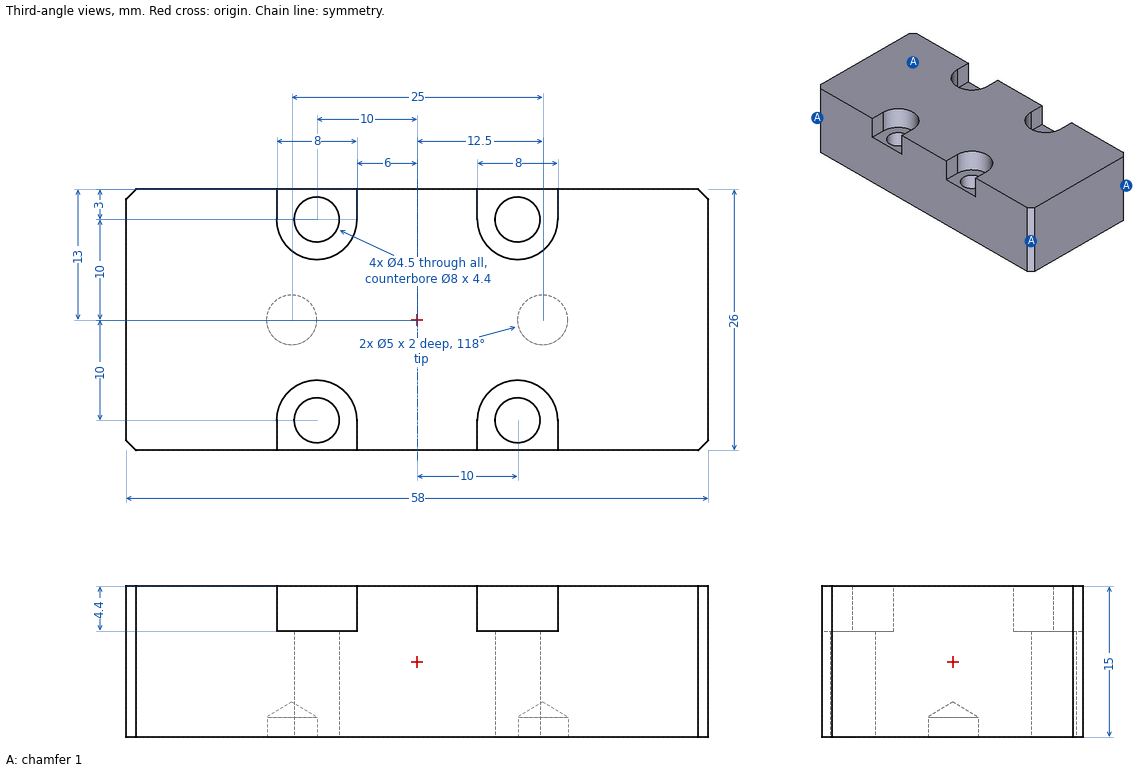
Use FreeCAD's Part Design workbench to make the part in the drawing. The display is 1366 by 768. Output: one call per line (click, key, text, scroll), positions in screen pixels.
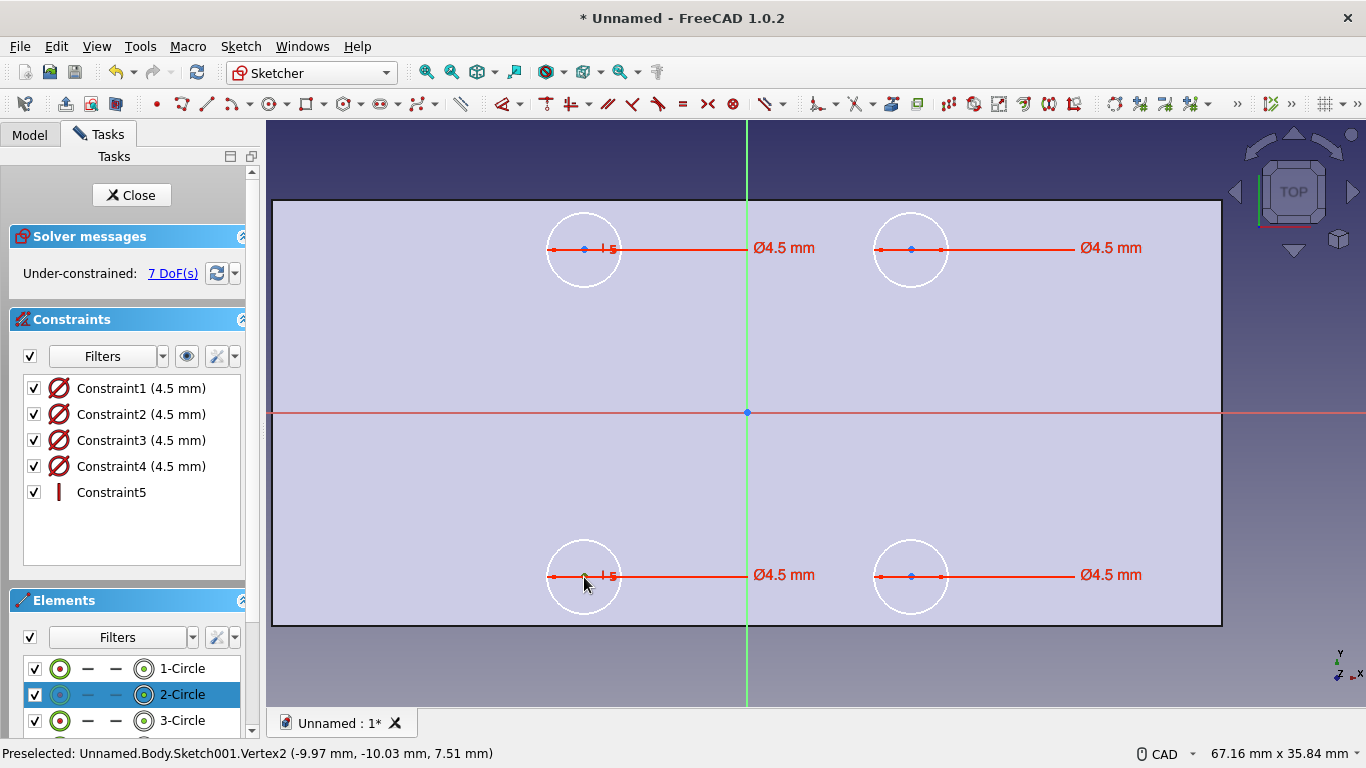
click(911, 577)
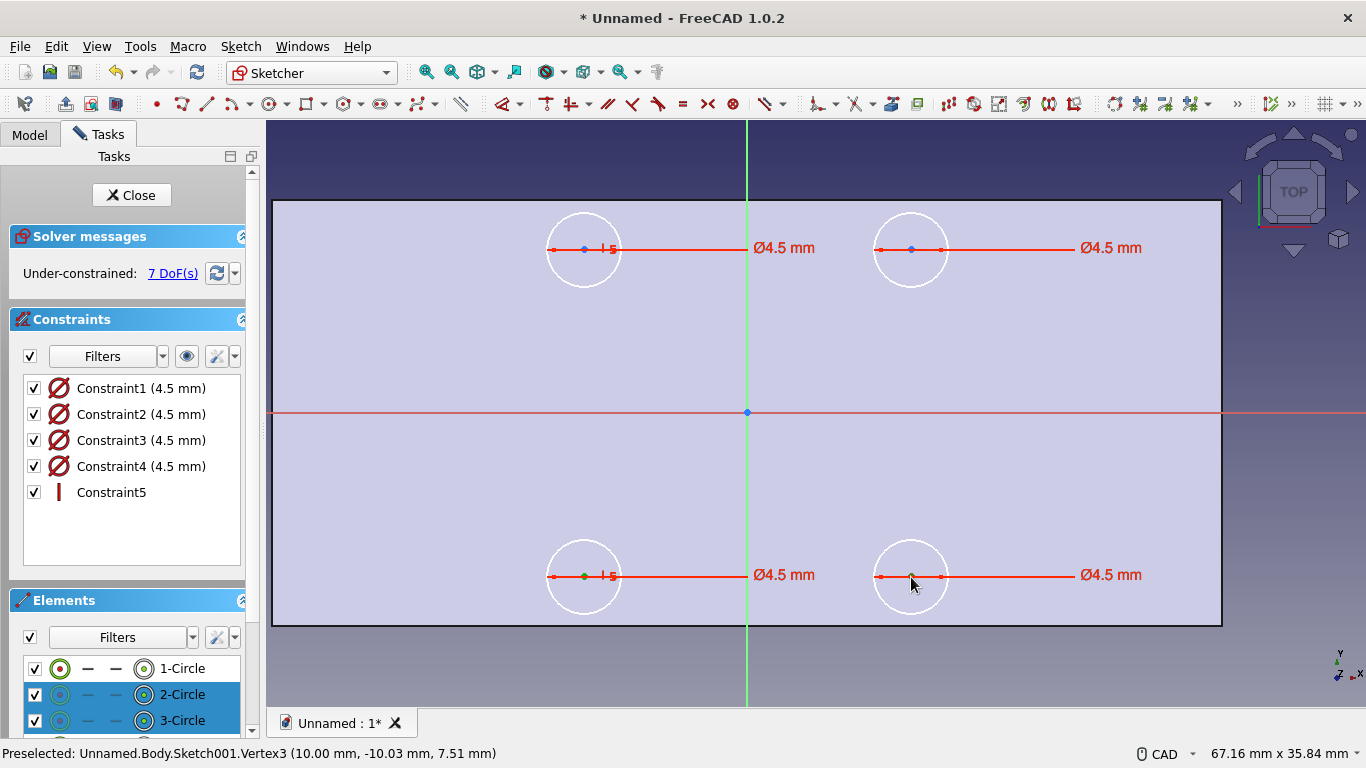
key(h)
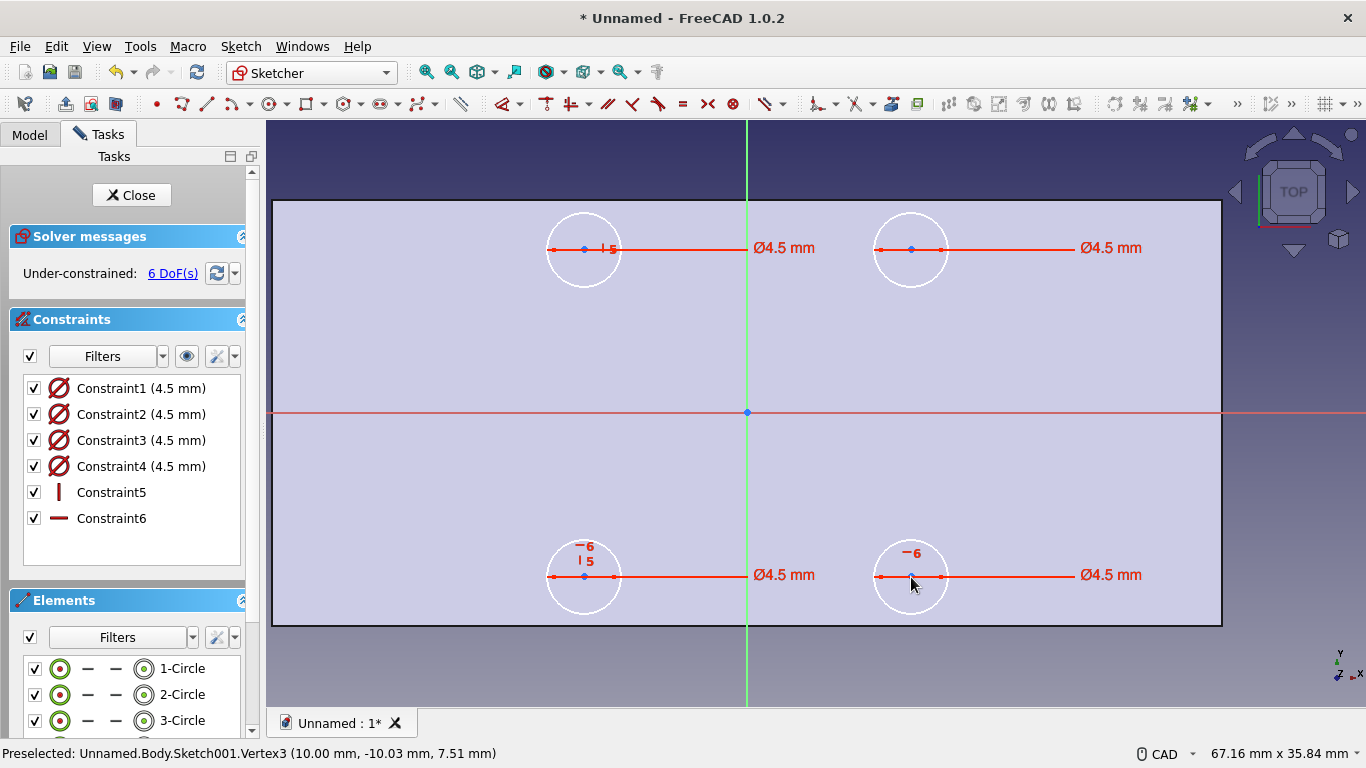
click(911, 577)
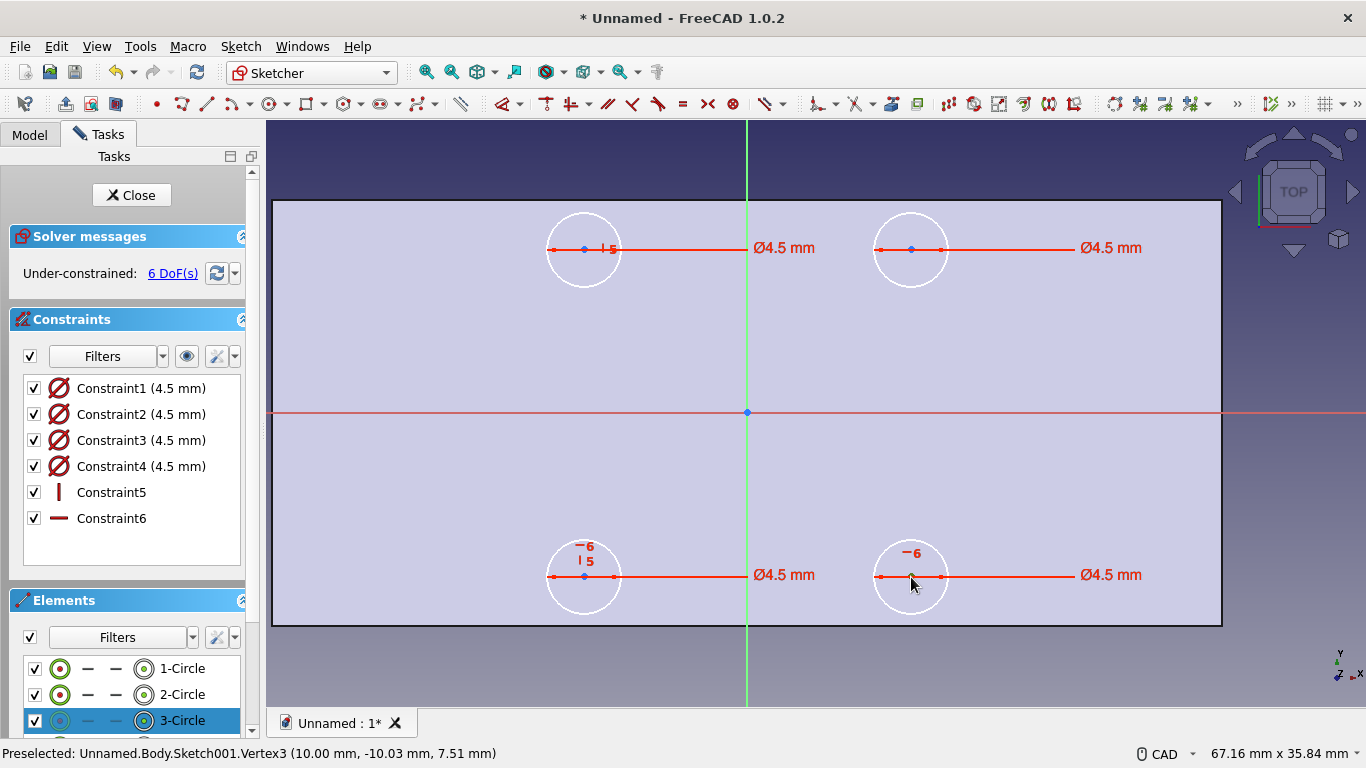
click(911, 250)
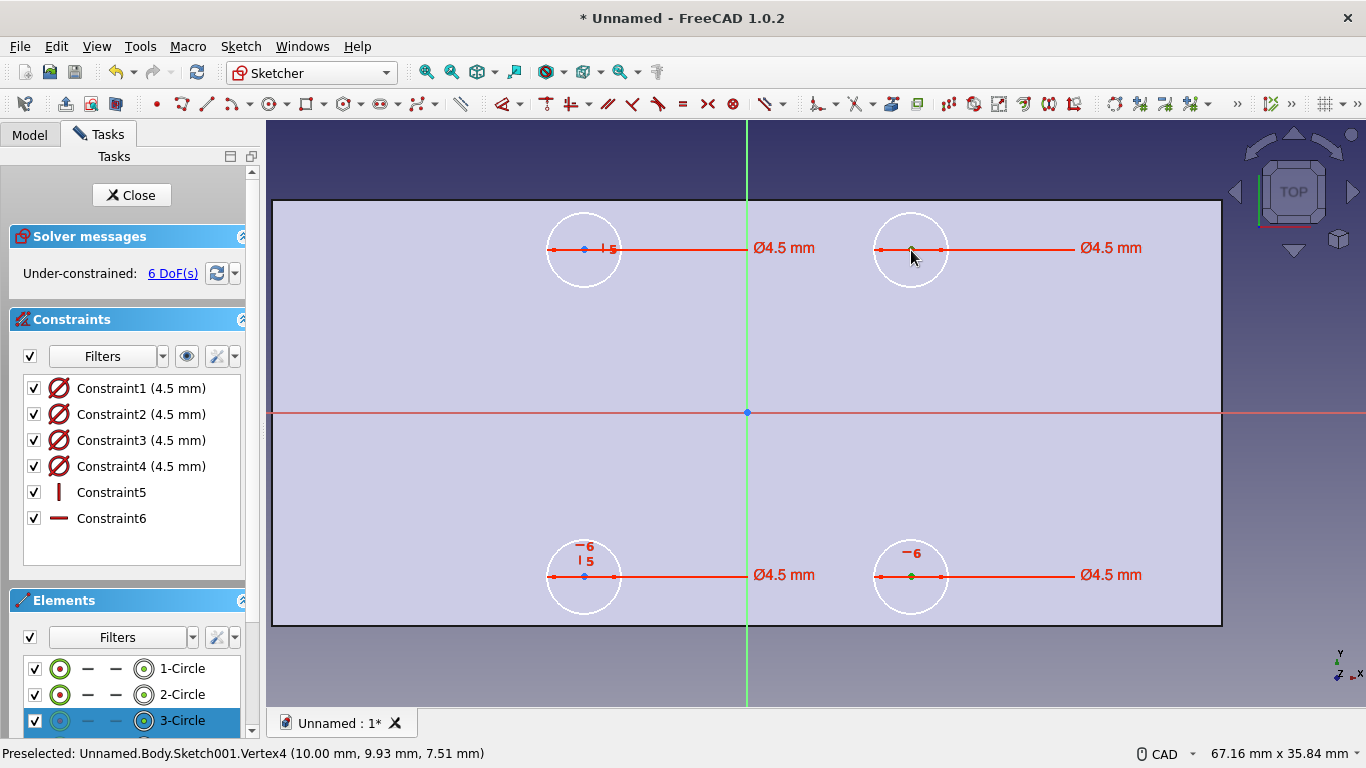
key(v)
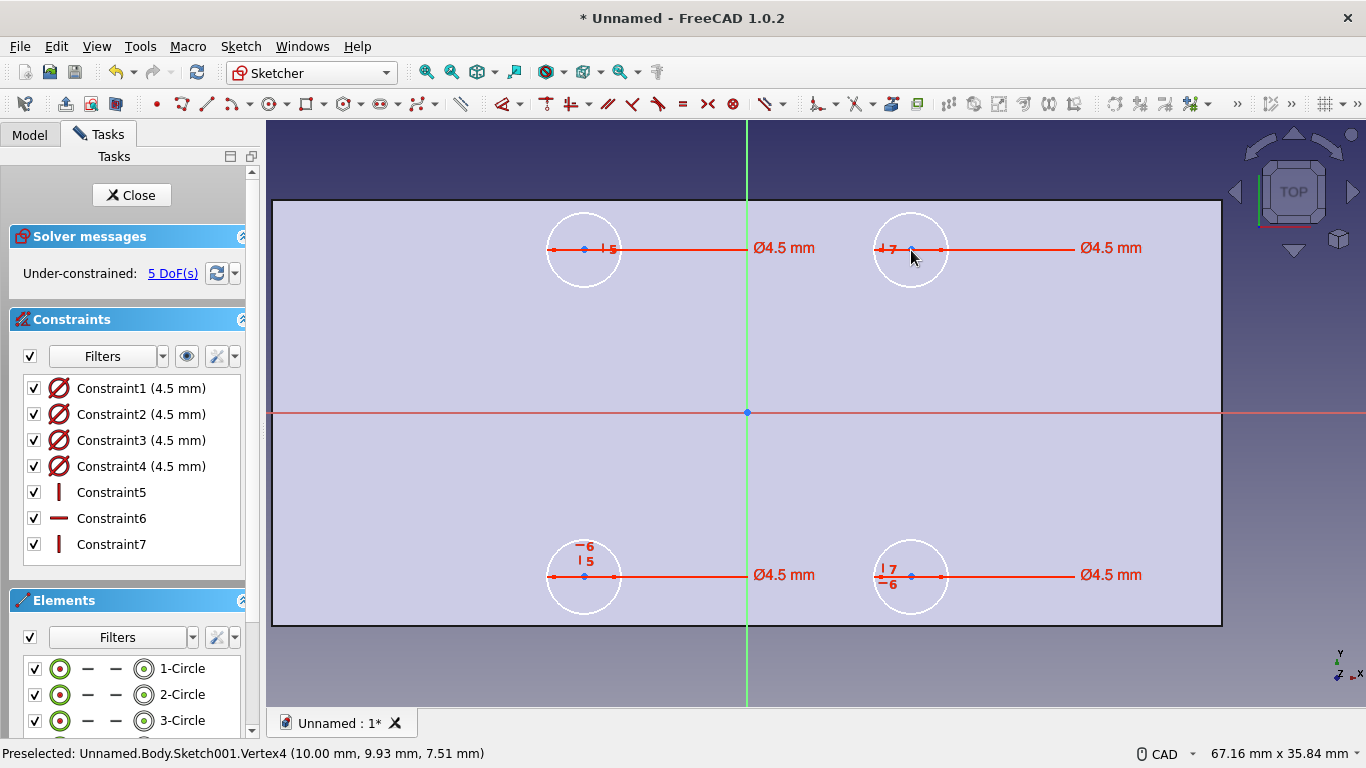
click(584, 250)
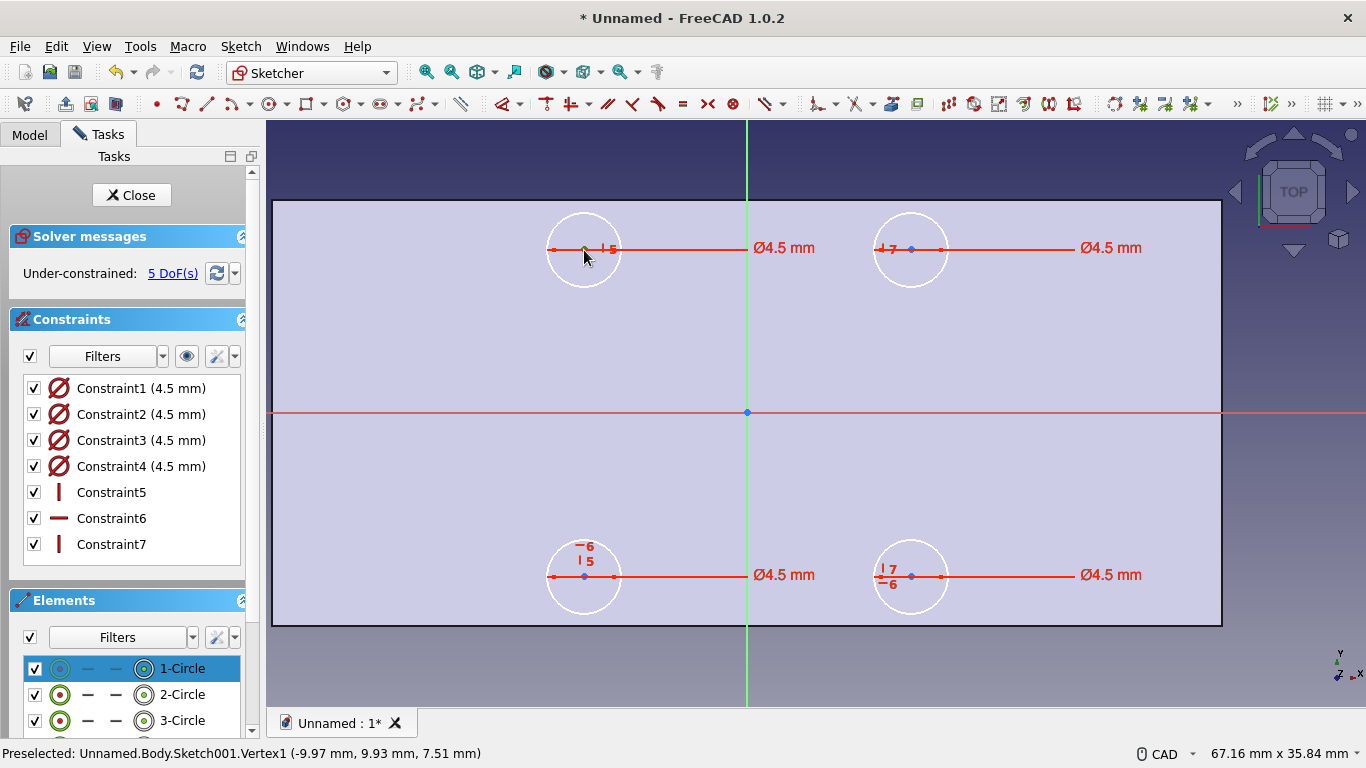
click(911, 250)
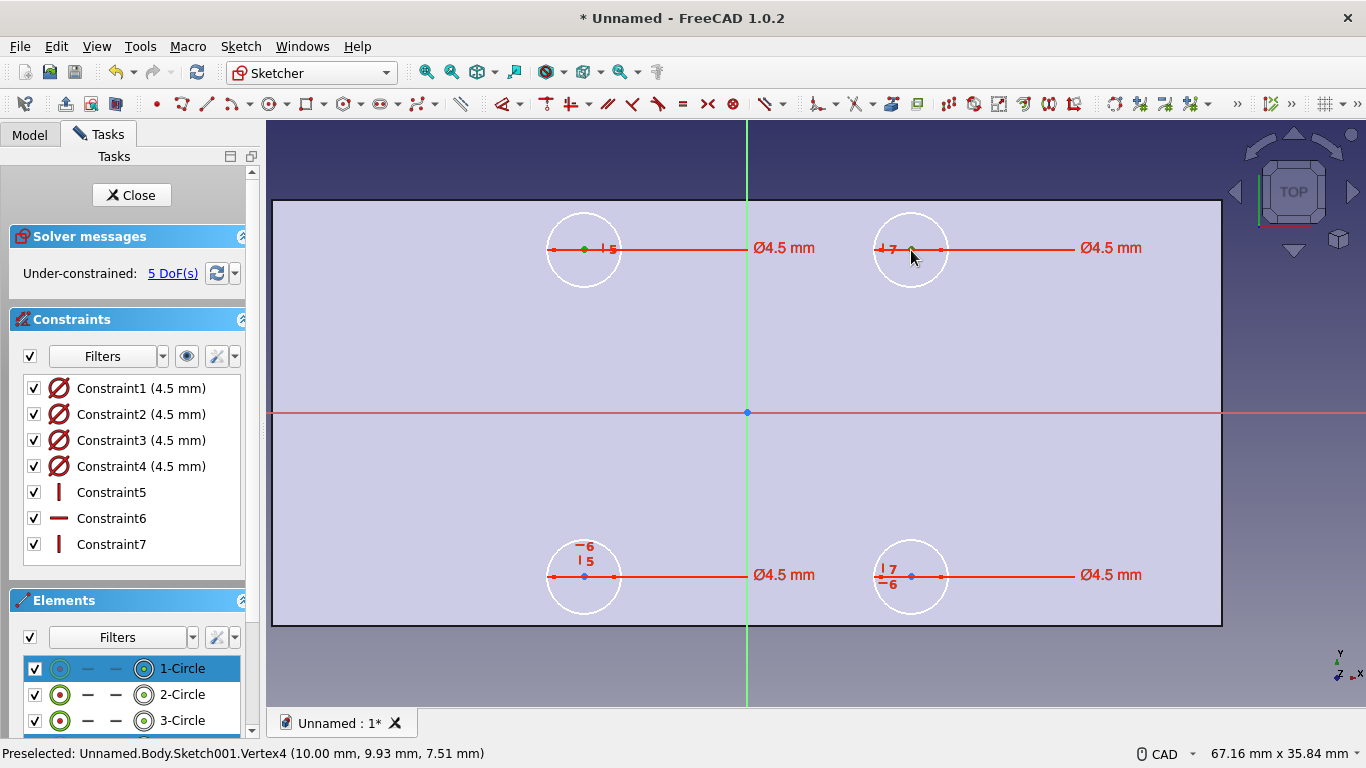
key(h)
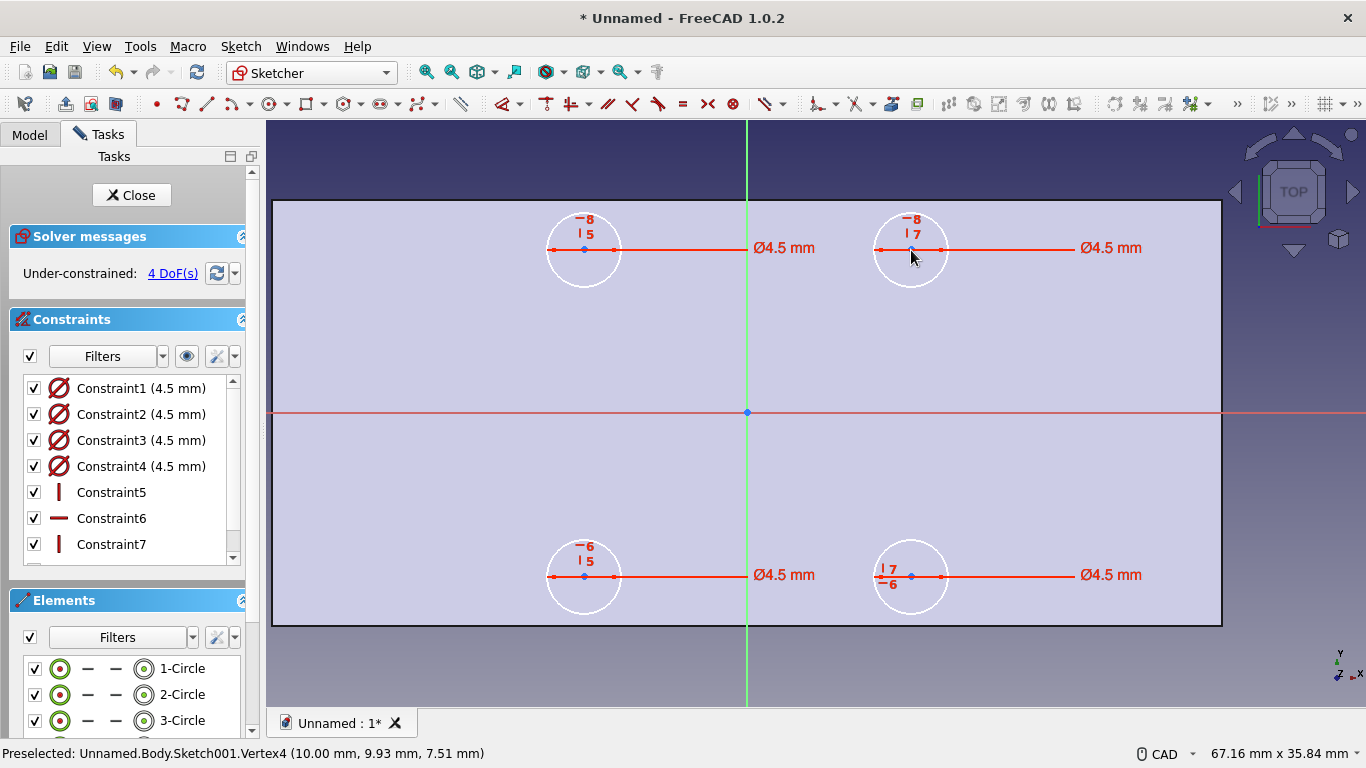
click(584, 250)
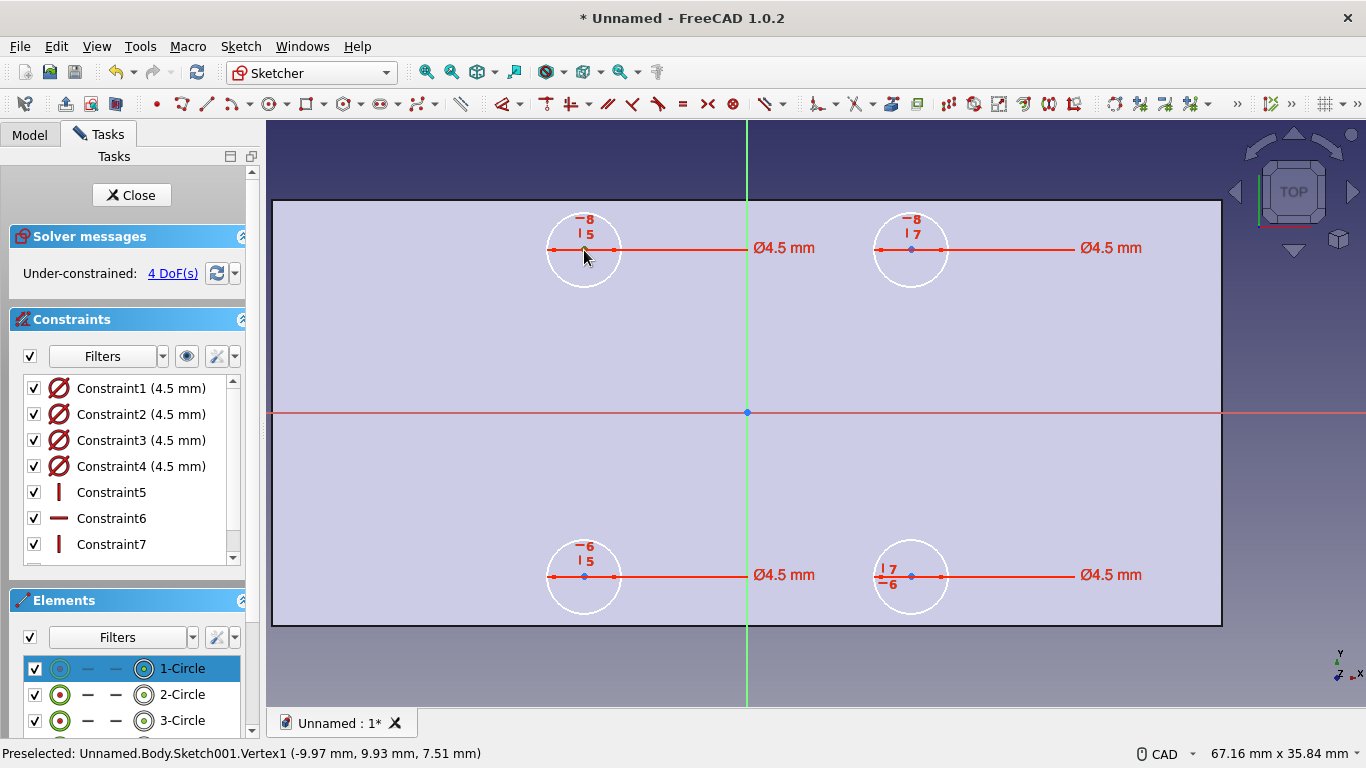
key(l)